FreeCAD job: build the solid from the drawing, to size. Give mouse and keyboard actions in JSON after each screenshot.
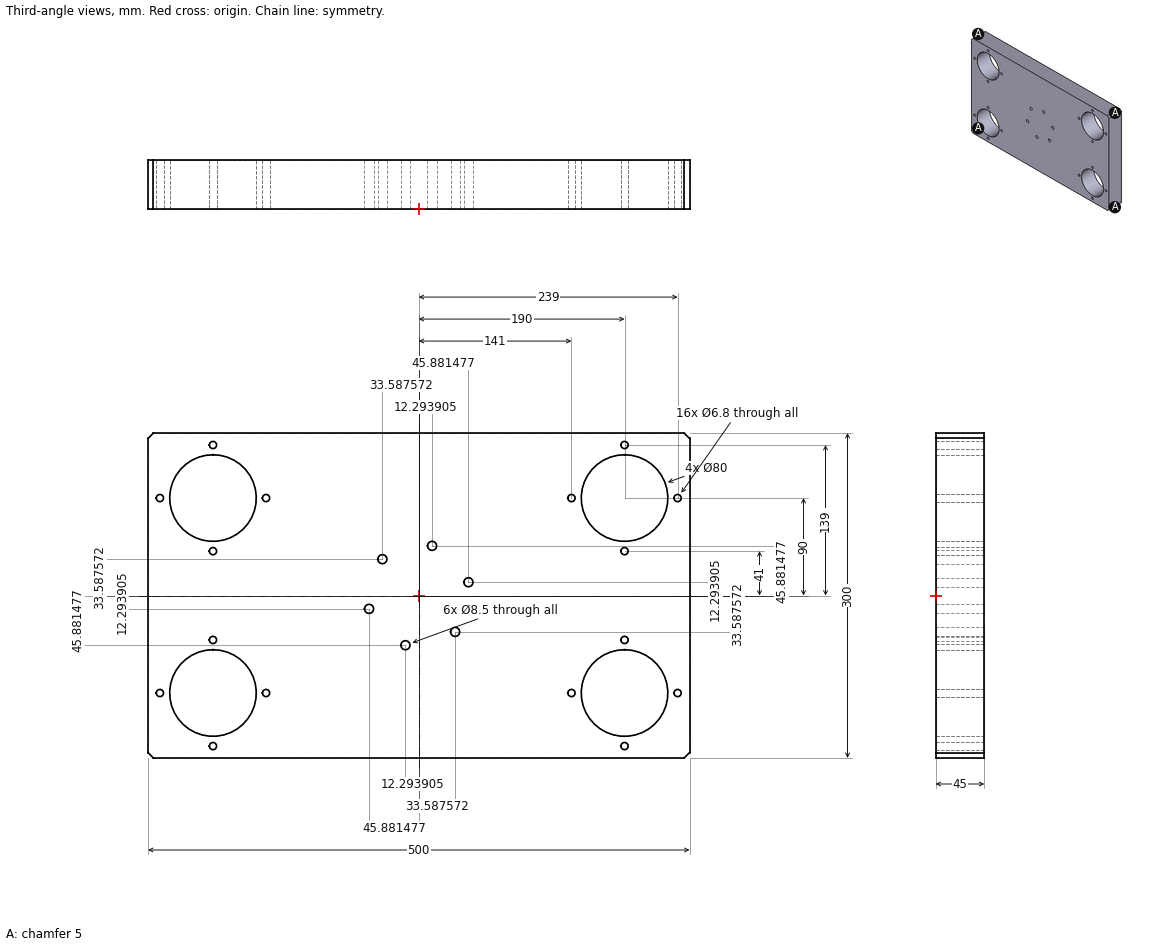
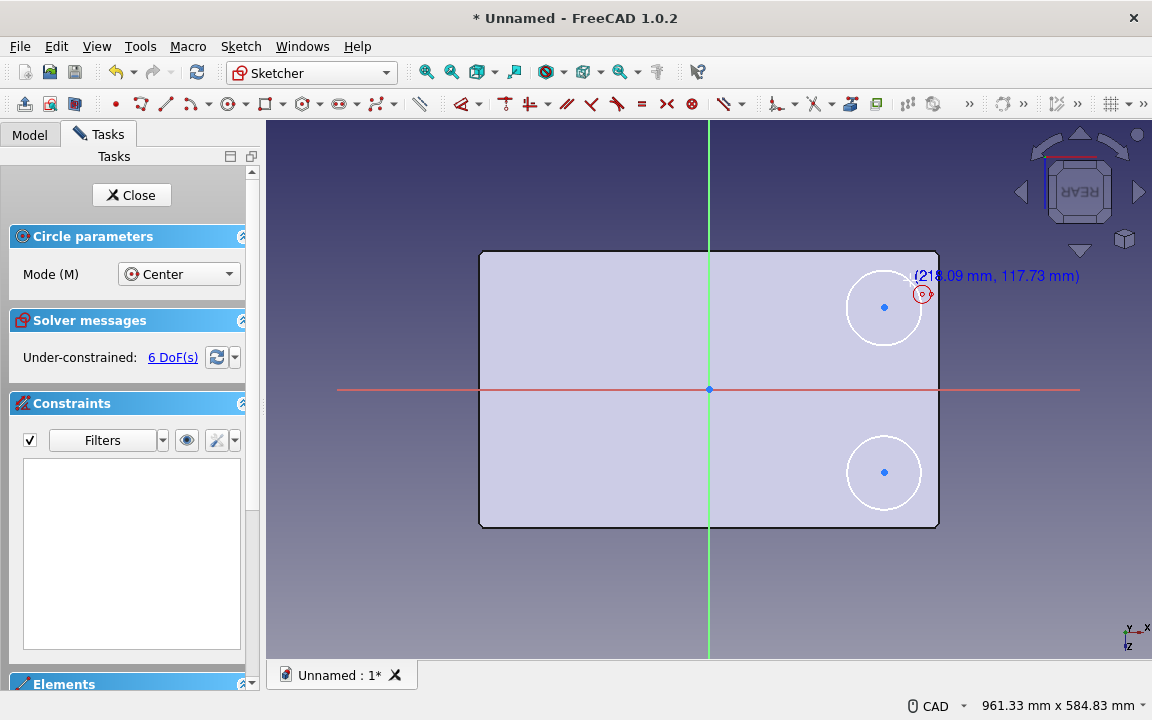
{"action": "left_click", "coordinate": [534, 307]}
{"action": "left_click", "coordinate": [560, 280]}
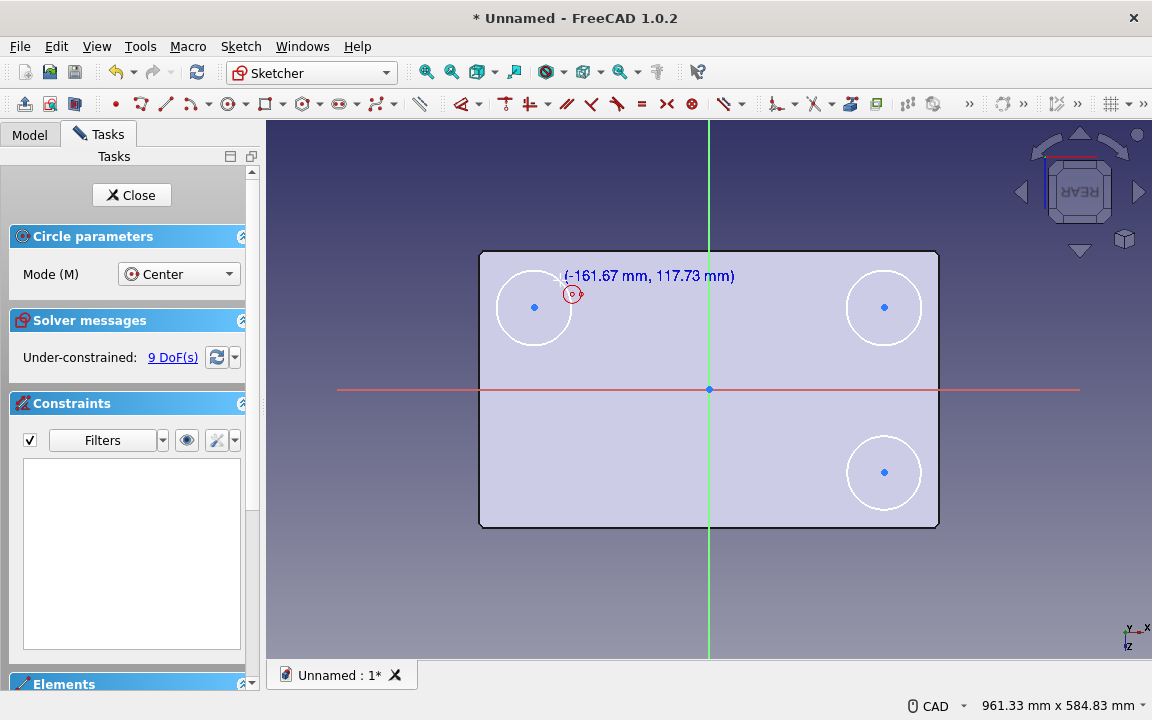
{"action": "left_click", "coordinate": [534, 472]}
{"action": "left_click", "coordinate": [560, 446]}
{"action": "key", "text": "Escape"}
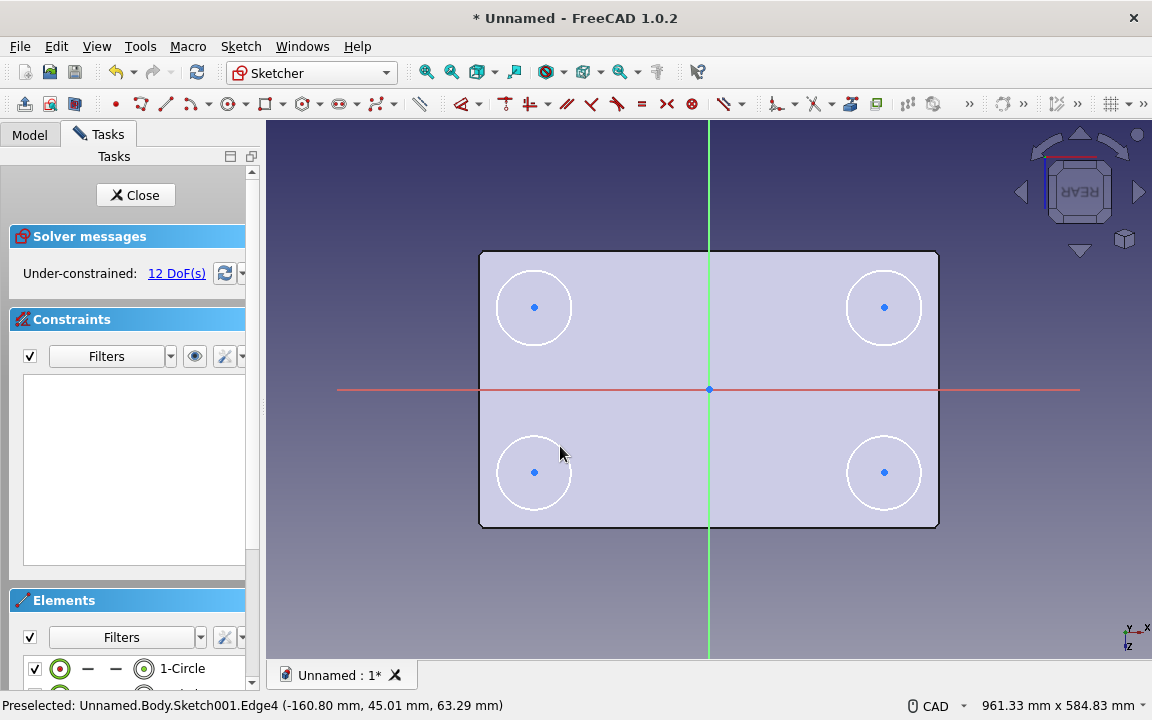
{"action": "left_click", "coordinate": [910, 447]}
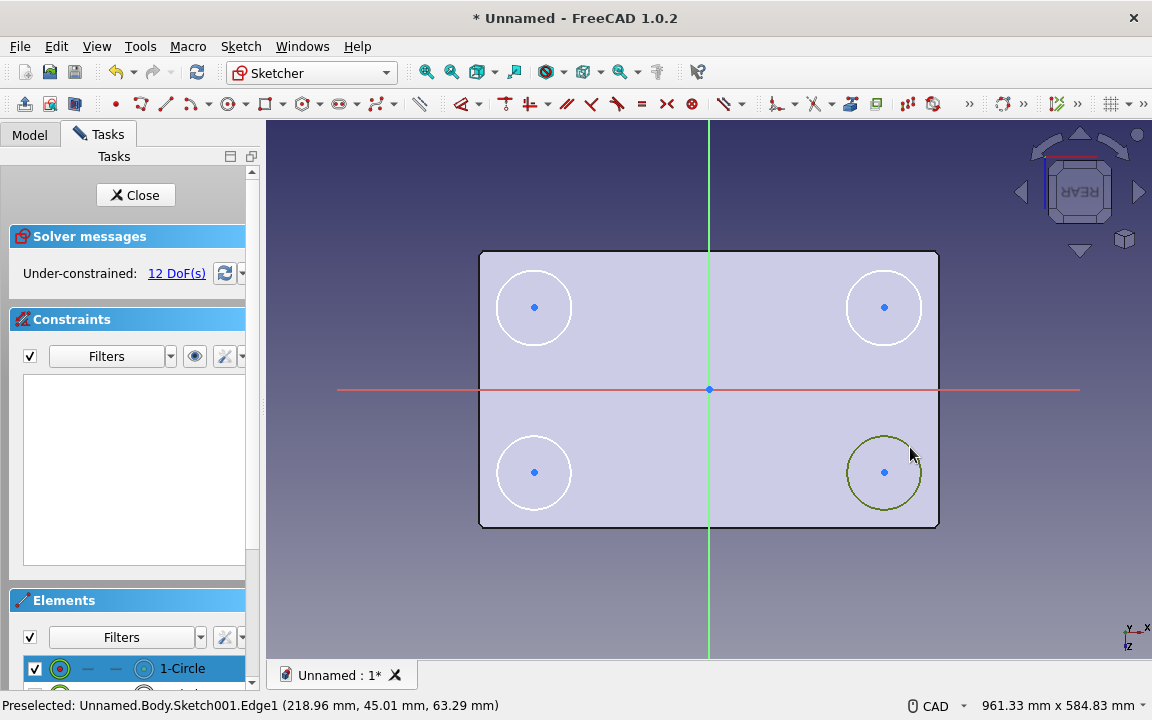
{"action": "left_click", "coordinate": [910, 281]}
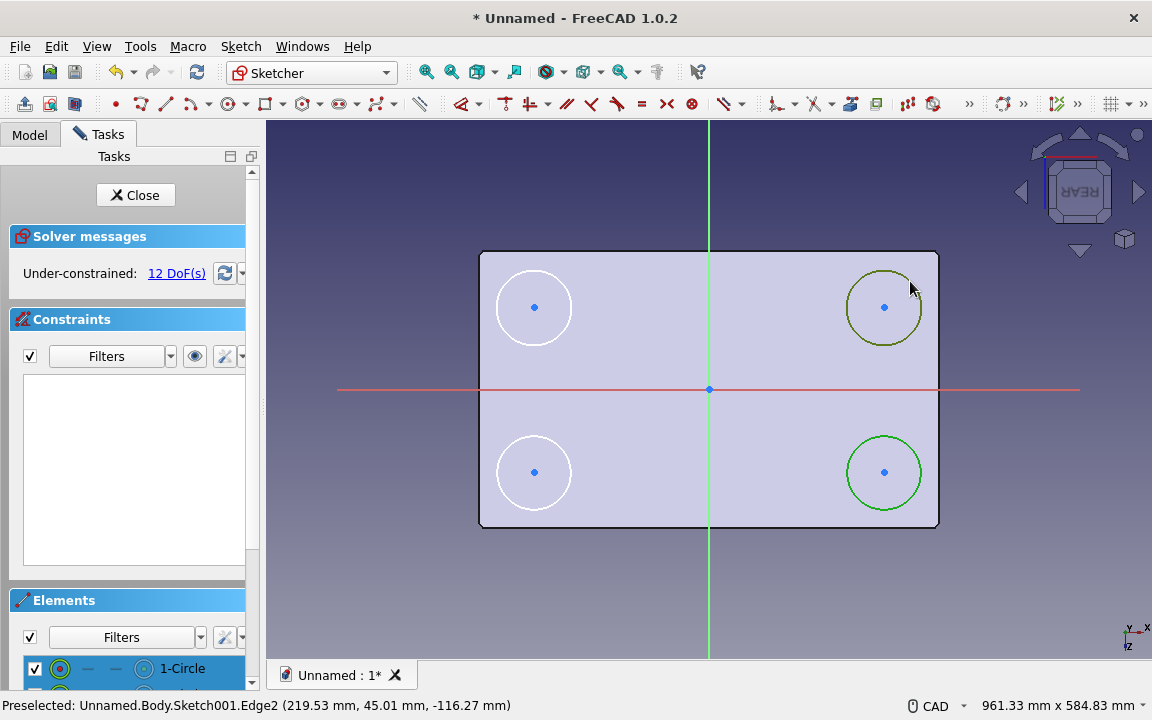
{"action": "left_click", "coordinate": [560, 281]}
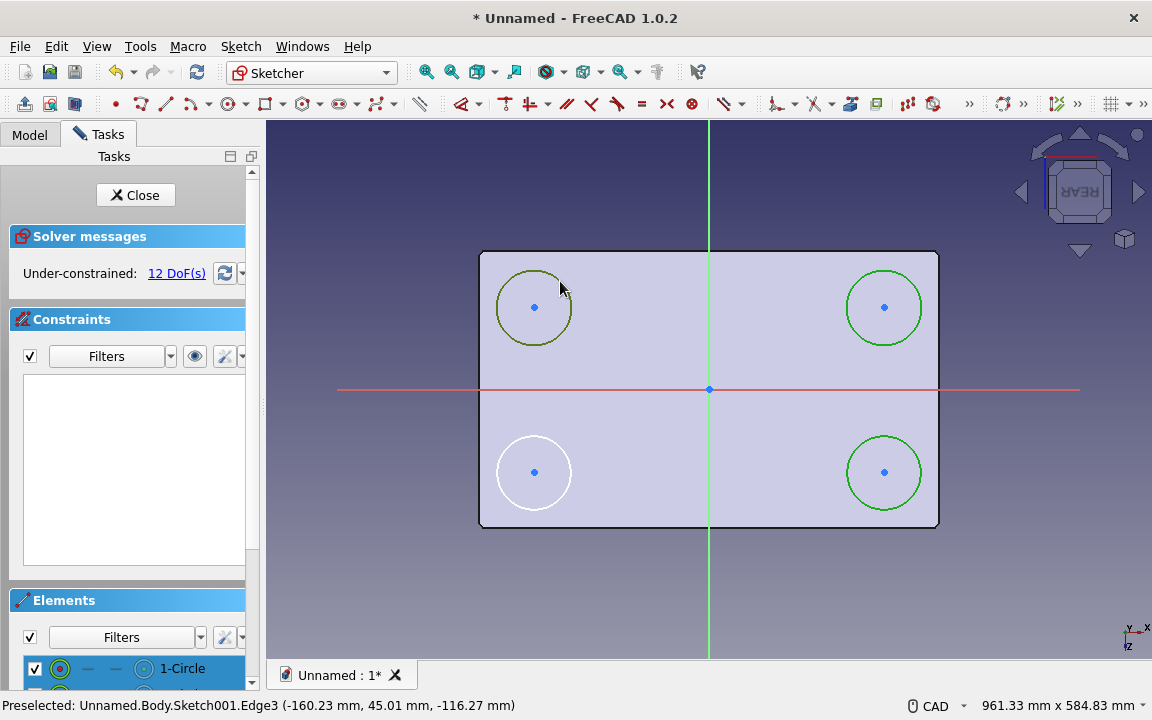
{"action": "left_click", "coordinate": [560, 447]}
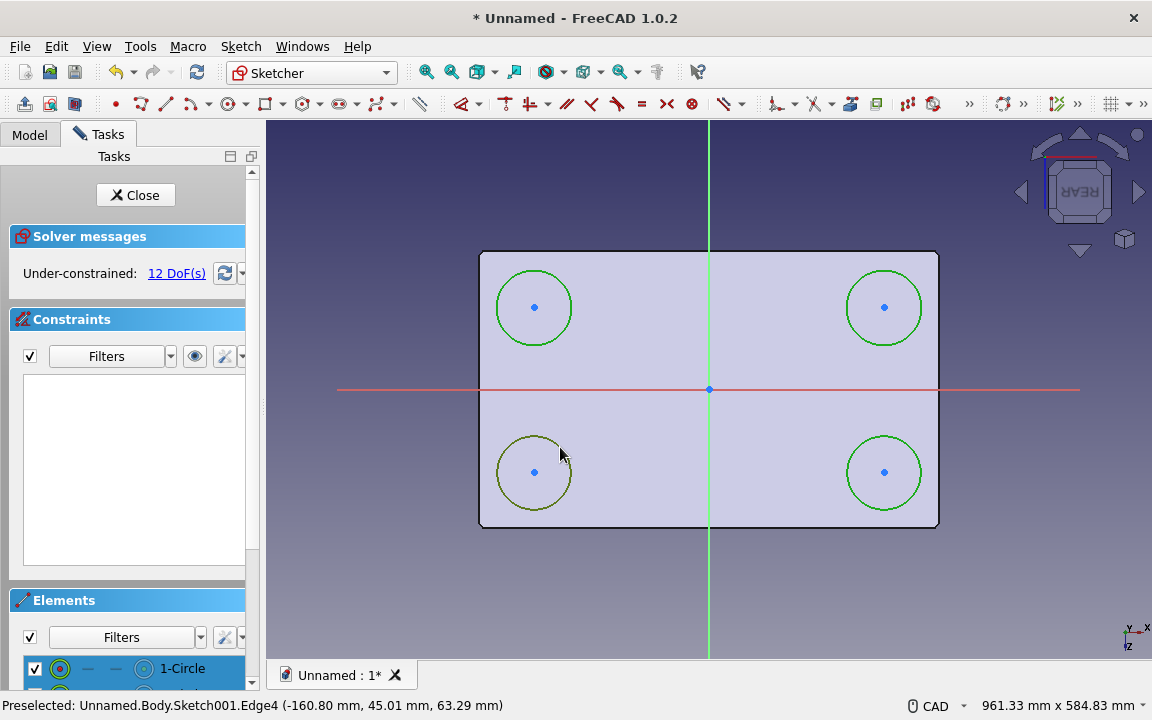
{"action": "left_click", "coordinate": [642, 104]}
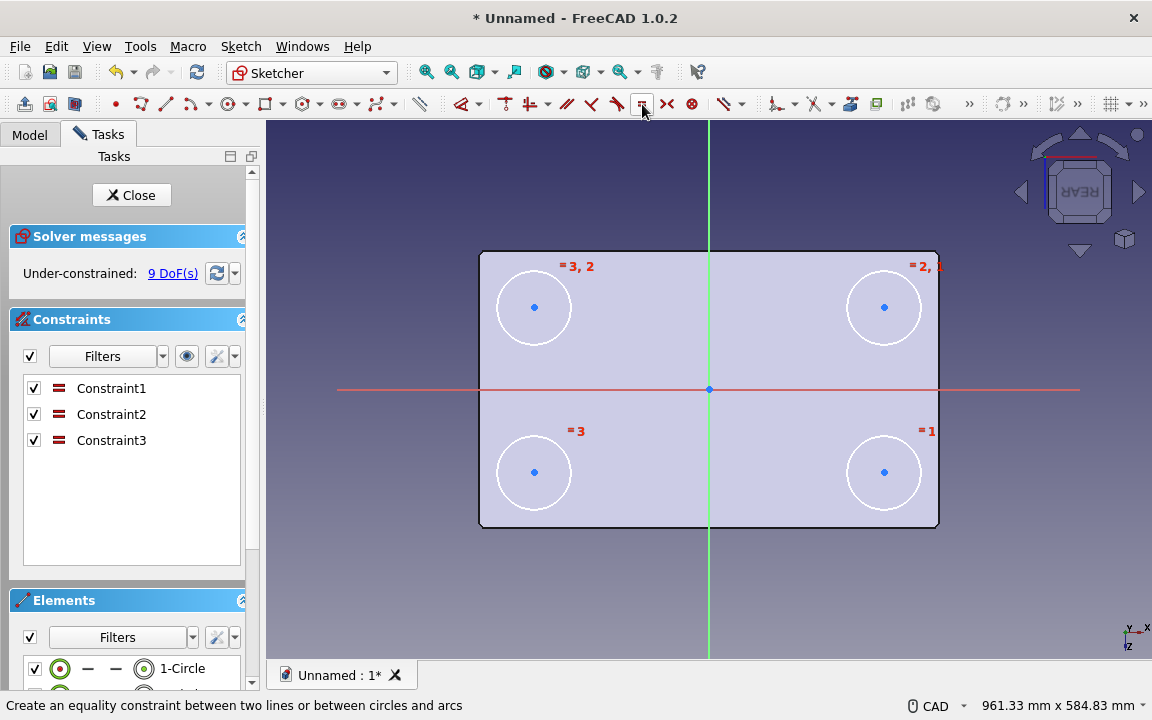
{"action": "left_click", "coordinate": [884, 473]}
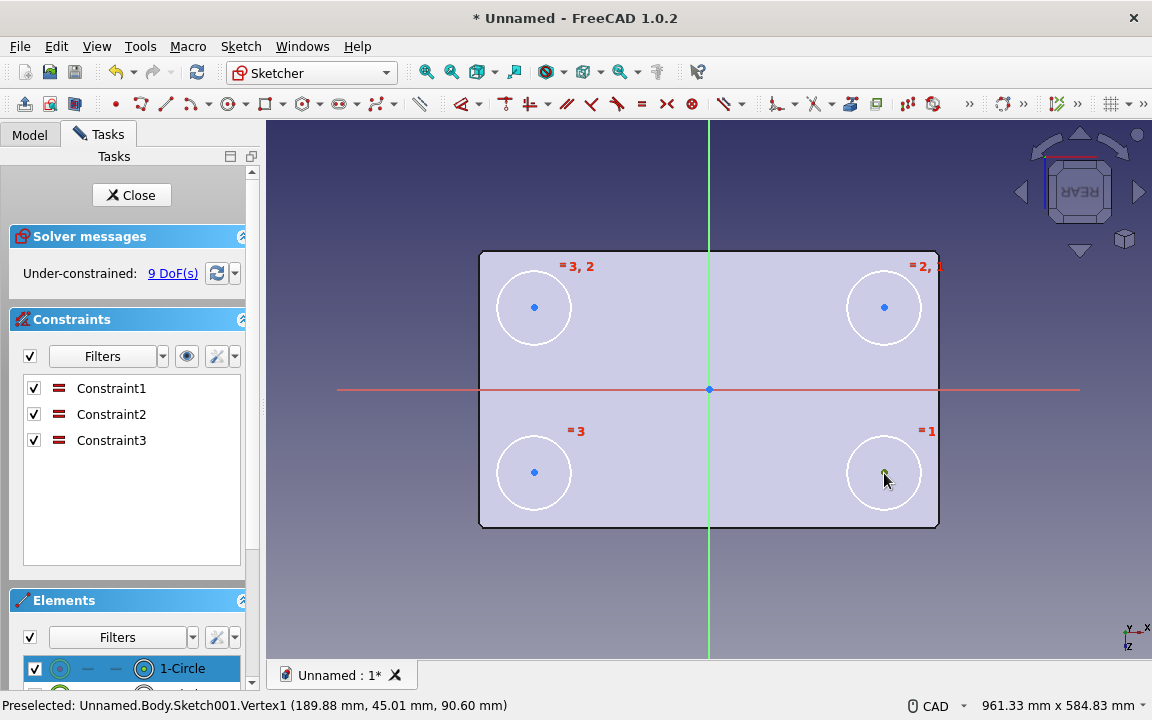
{"action": "left_click", "coordinate": [884, 308]}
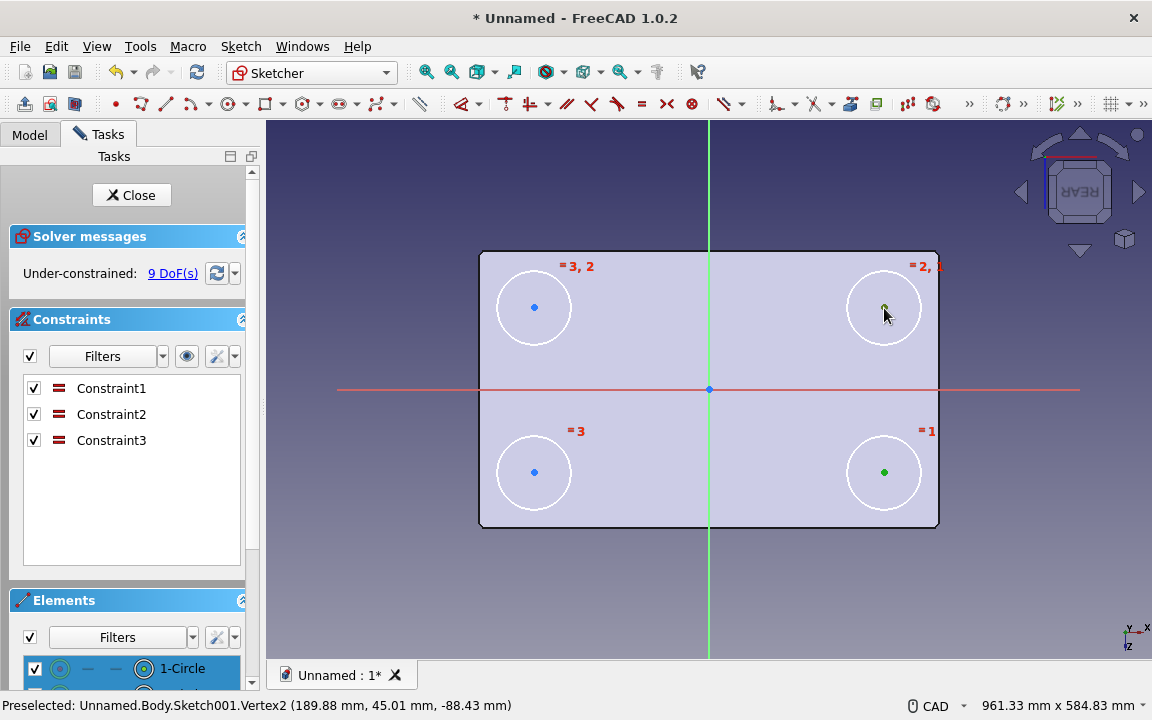
{"action": "left_click", "coordinate": [344, 389]}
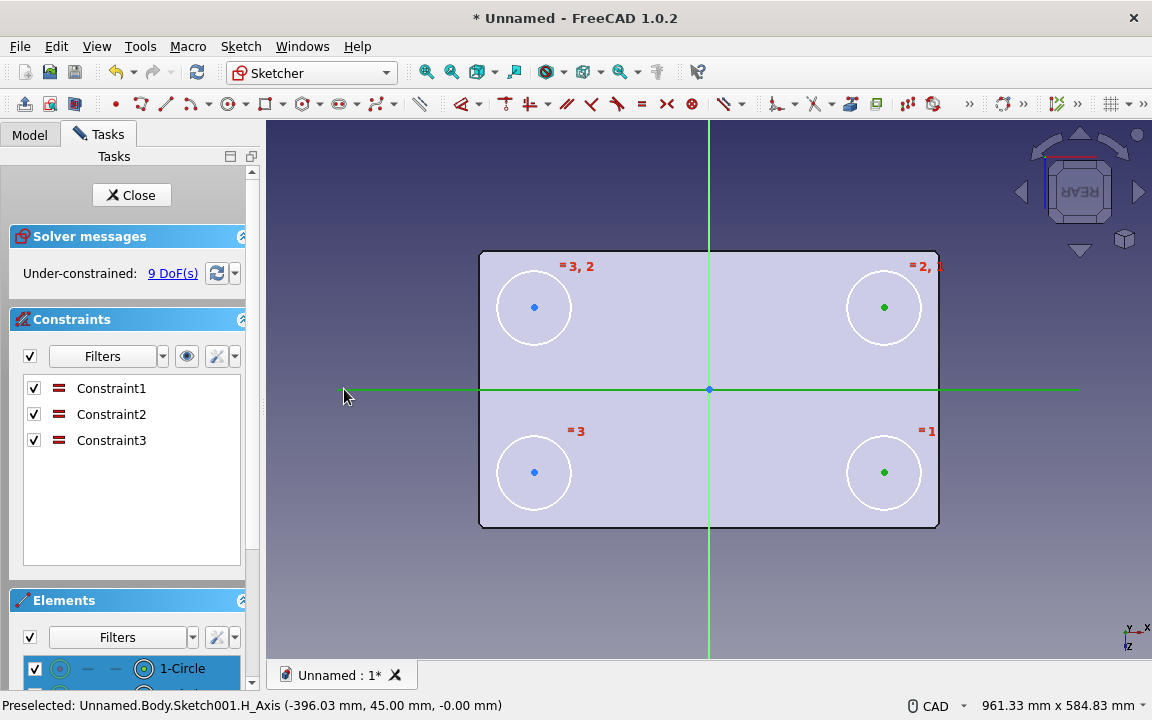
{"action": "left_click", "coordinate": [667, 104]}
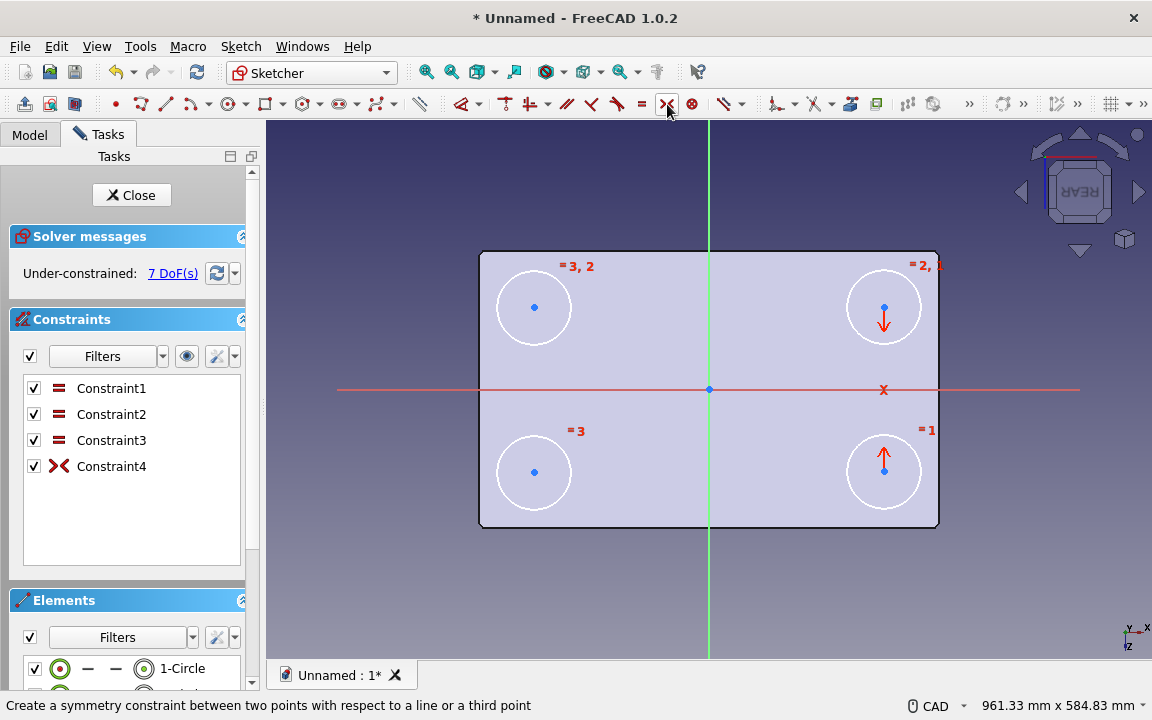
{"action": "left_click", "coordinate": [884, 307]}